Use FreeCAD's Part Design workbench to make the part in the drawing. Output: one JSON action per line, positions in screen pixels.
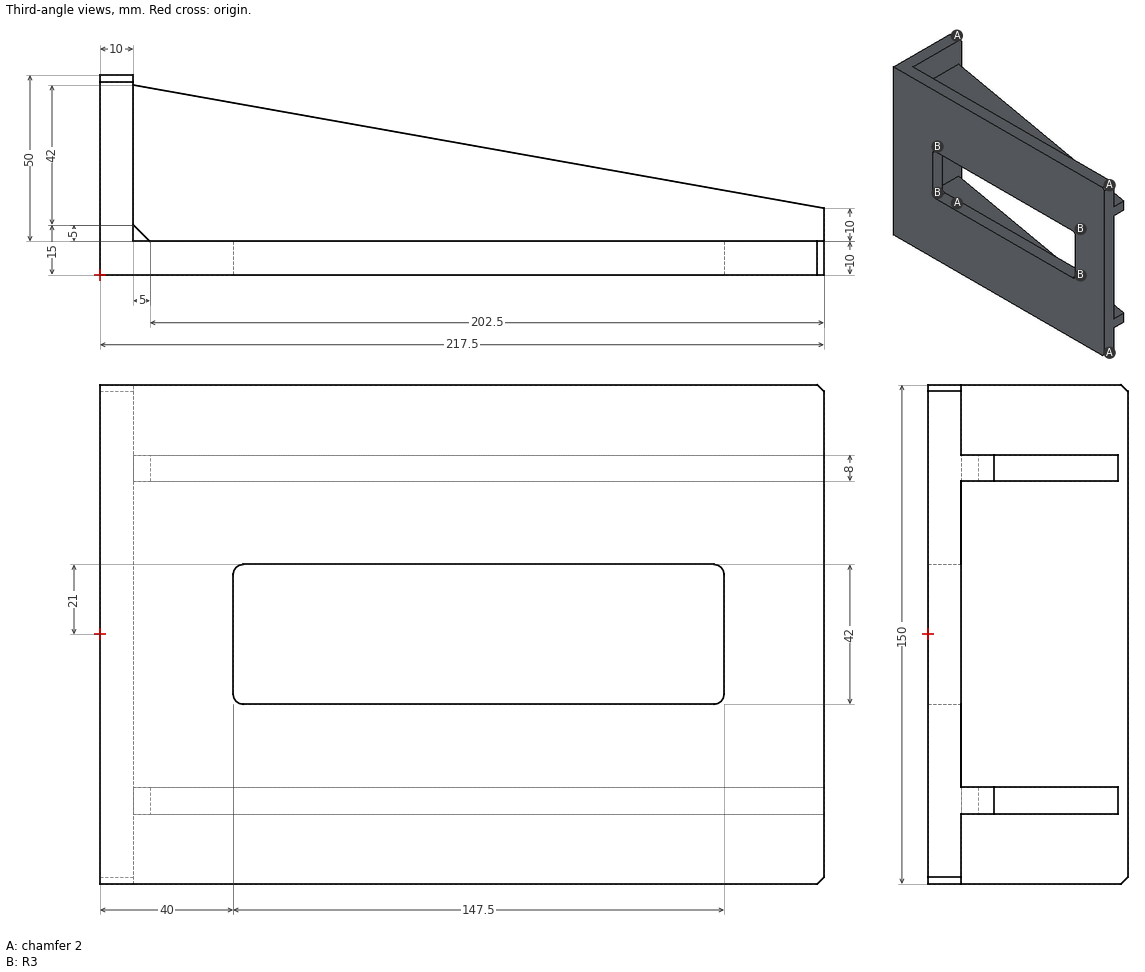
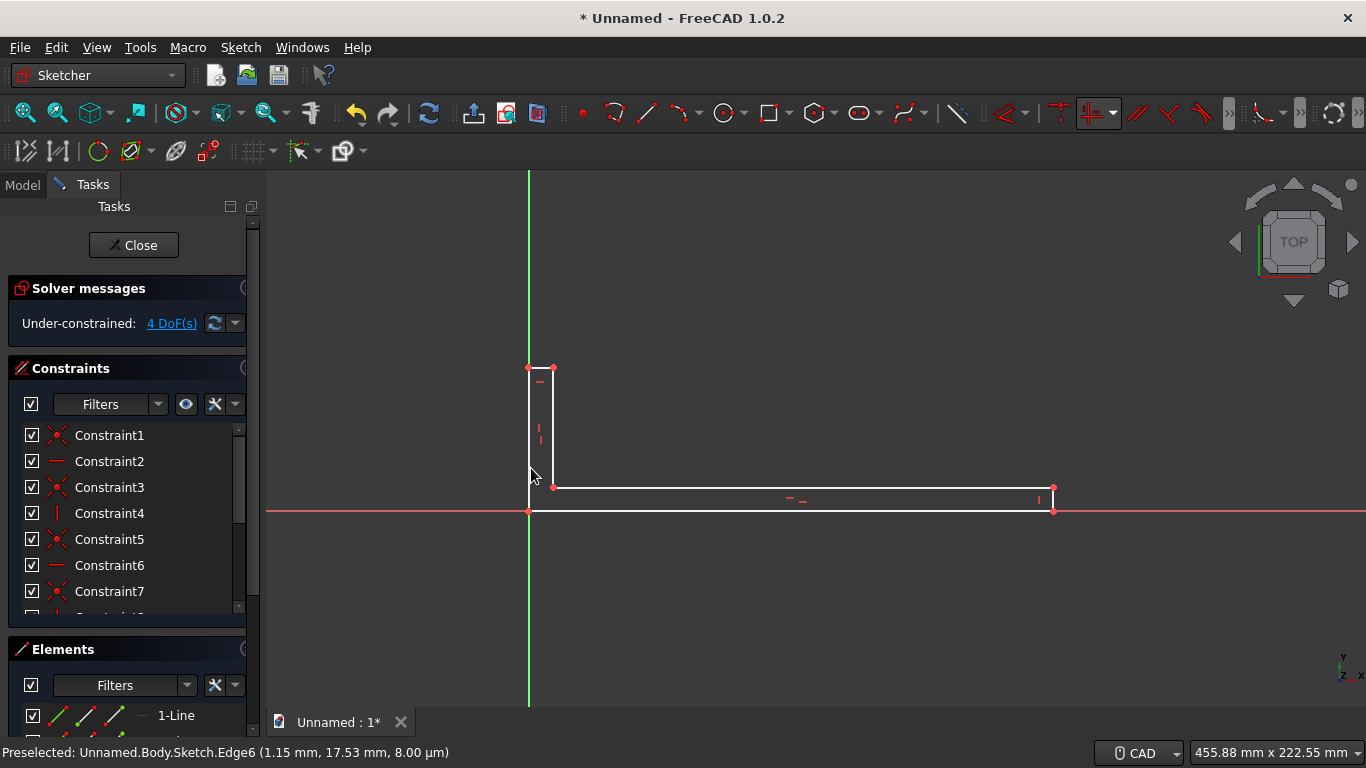
{"action": "left_click", "coordinate": [1004, 114]}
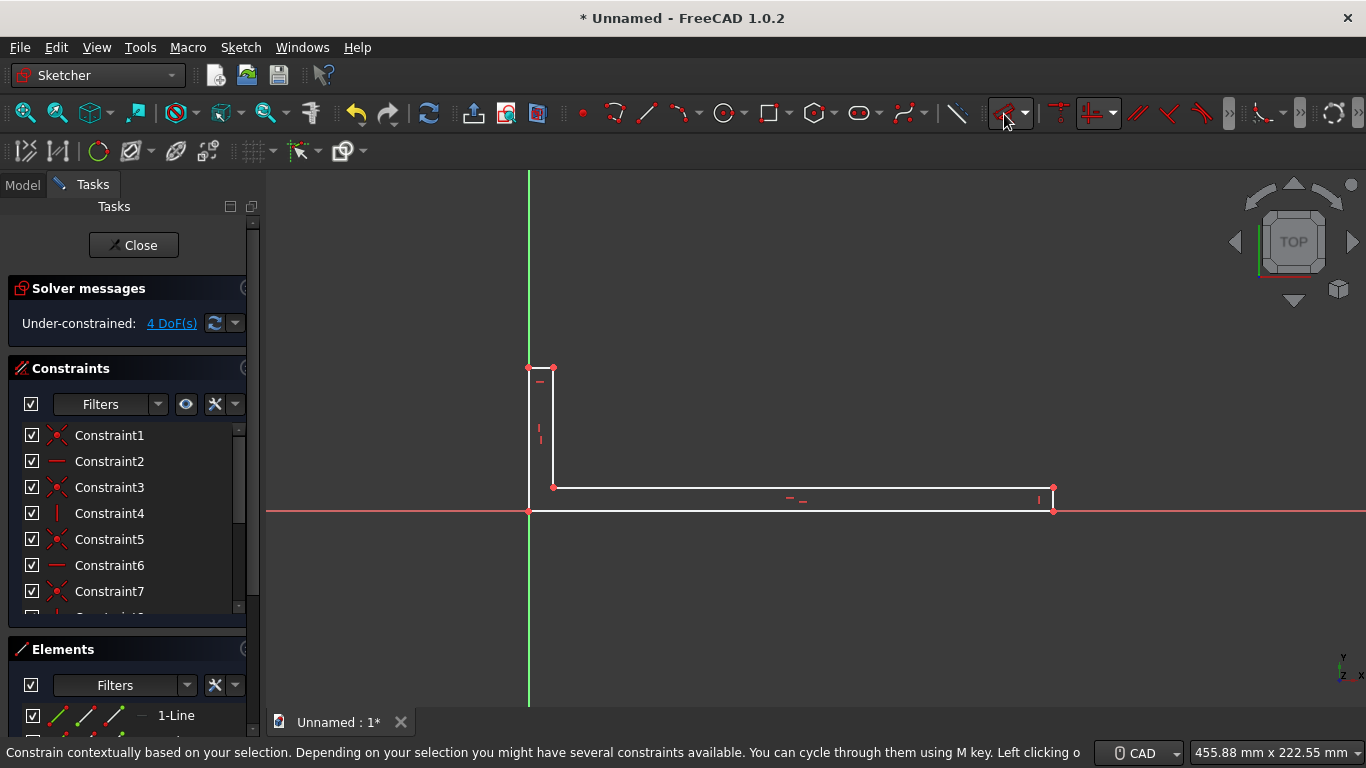
{"action": "scroll", "coordinate": [1053, 502], "scroll_direction": "up", "scroll_amount": 3}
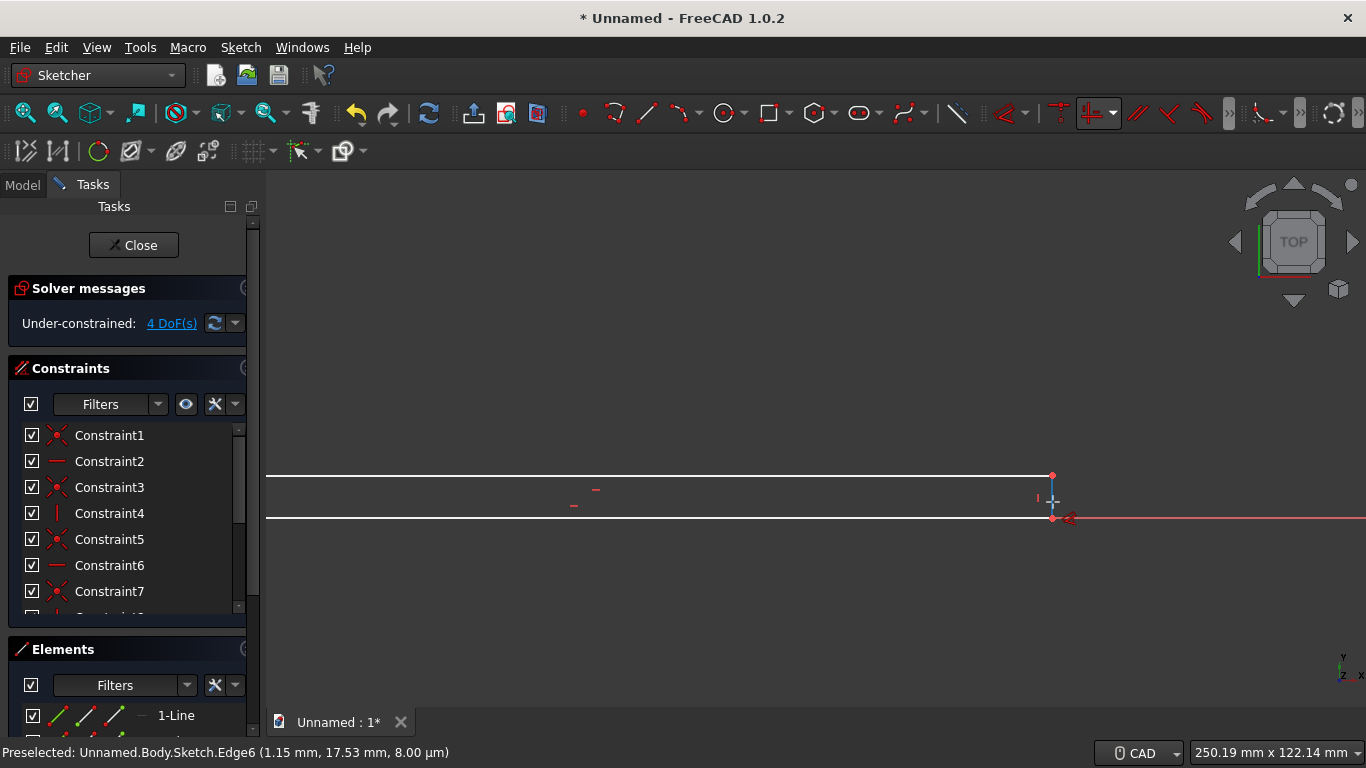
{"action": "left_click", "coordinate": [1052, 501]}
{"action": "left_click", "coordinate": [1086, 497]}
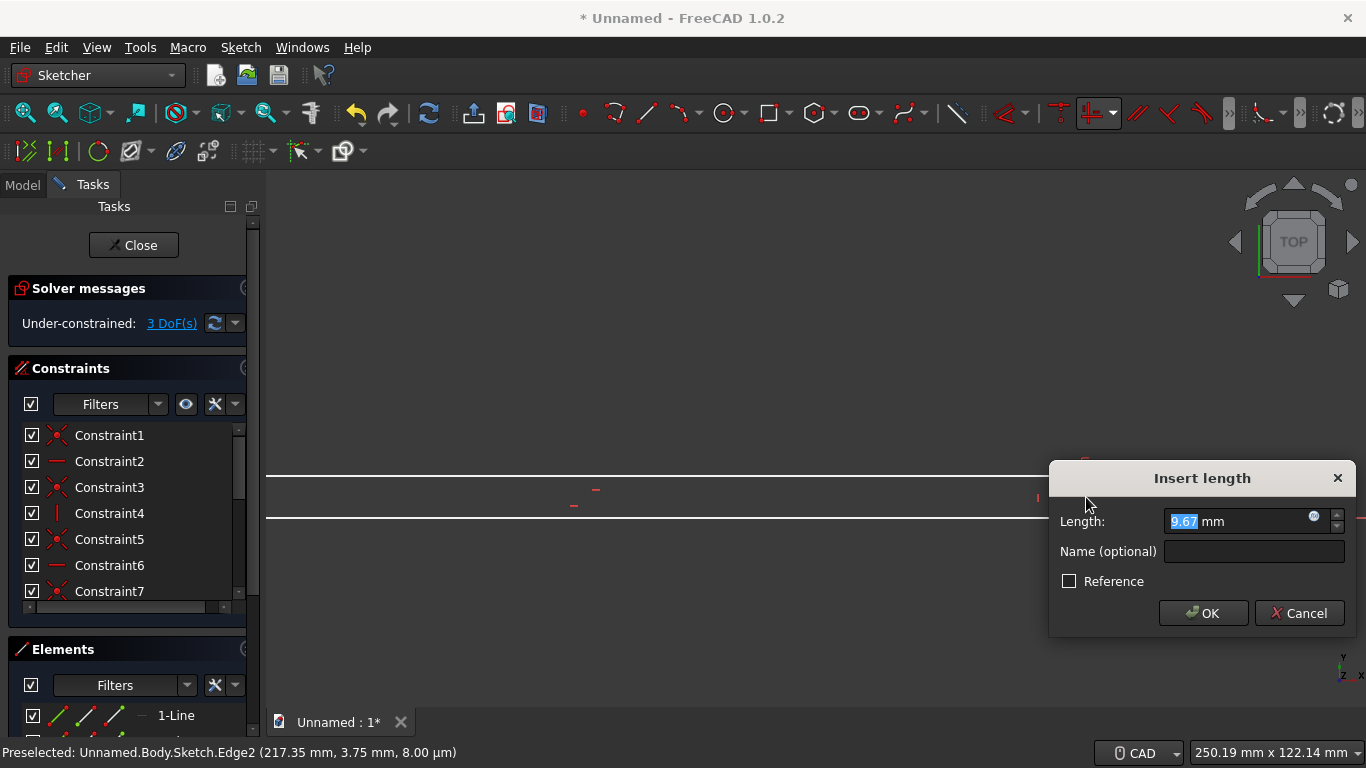
{"action": "type", "text": "10"}
{"action": "key", "text": "Return"}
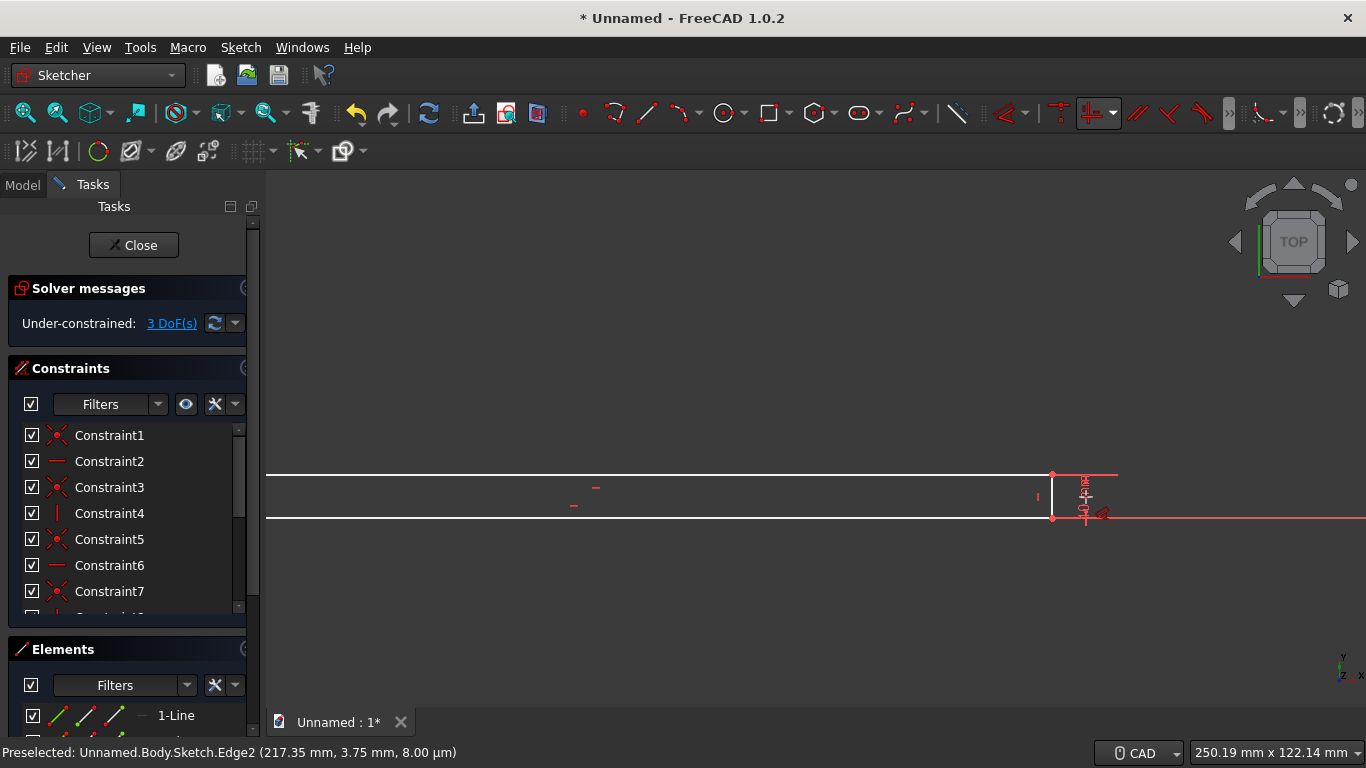
{"action": "scroll", "coordinate": [1098, 544], "scroll_direction": "down", "scroll_amount": 2}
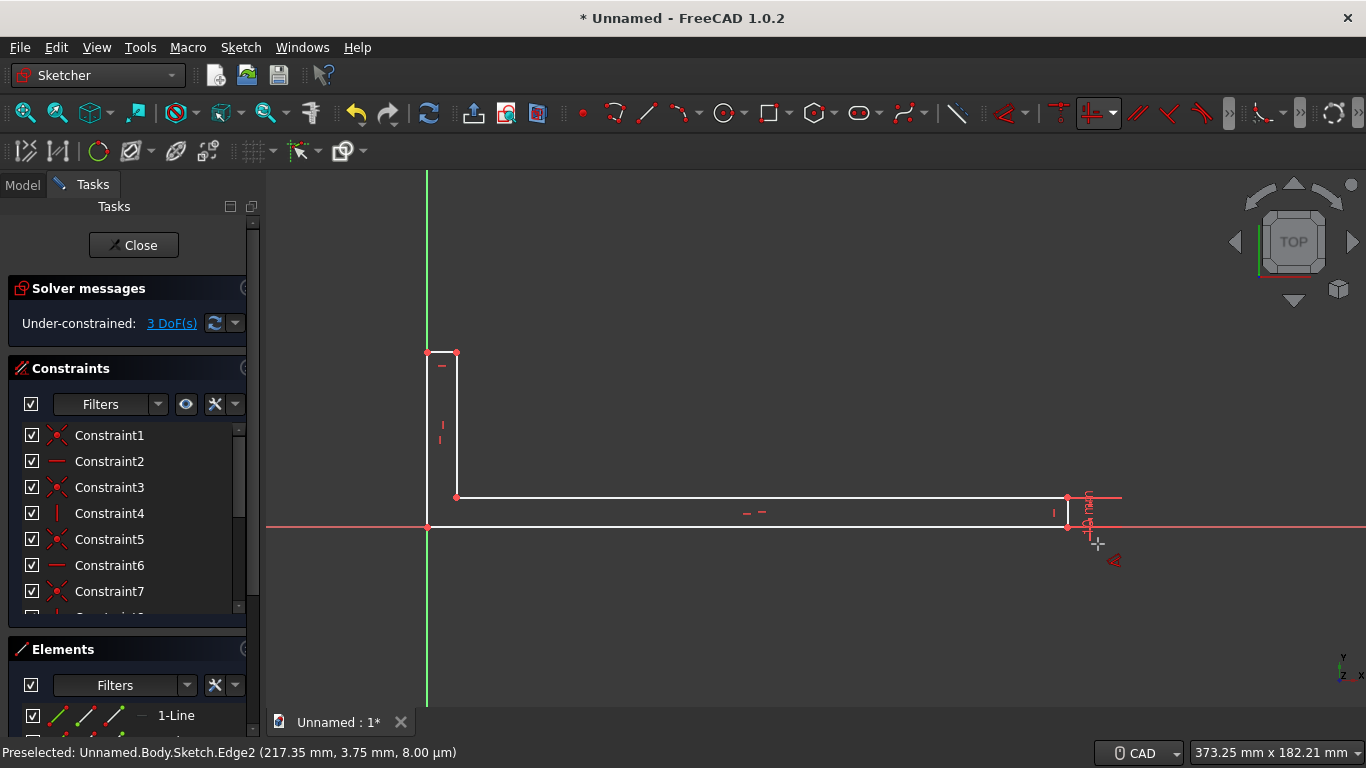
{"action": "left_click", "coordinate": [457, 454]}
{"action": "left_click", "coordinate": [491, 425]}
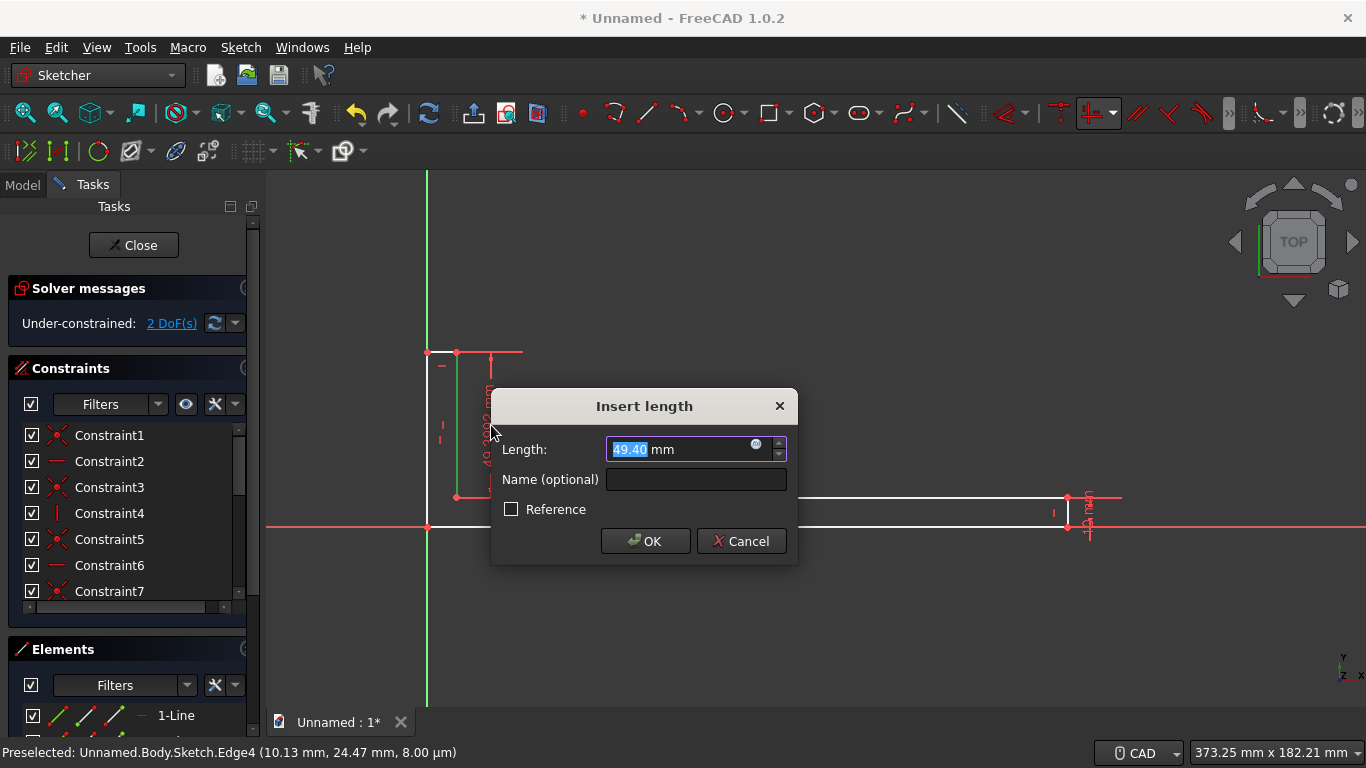
{"action": "type", "text": "50"}
{"action": "key", "text": "Return"}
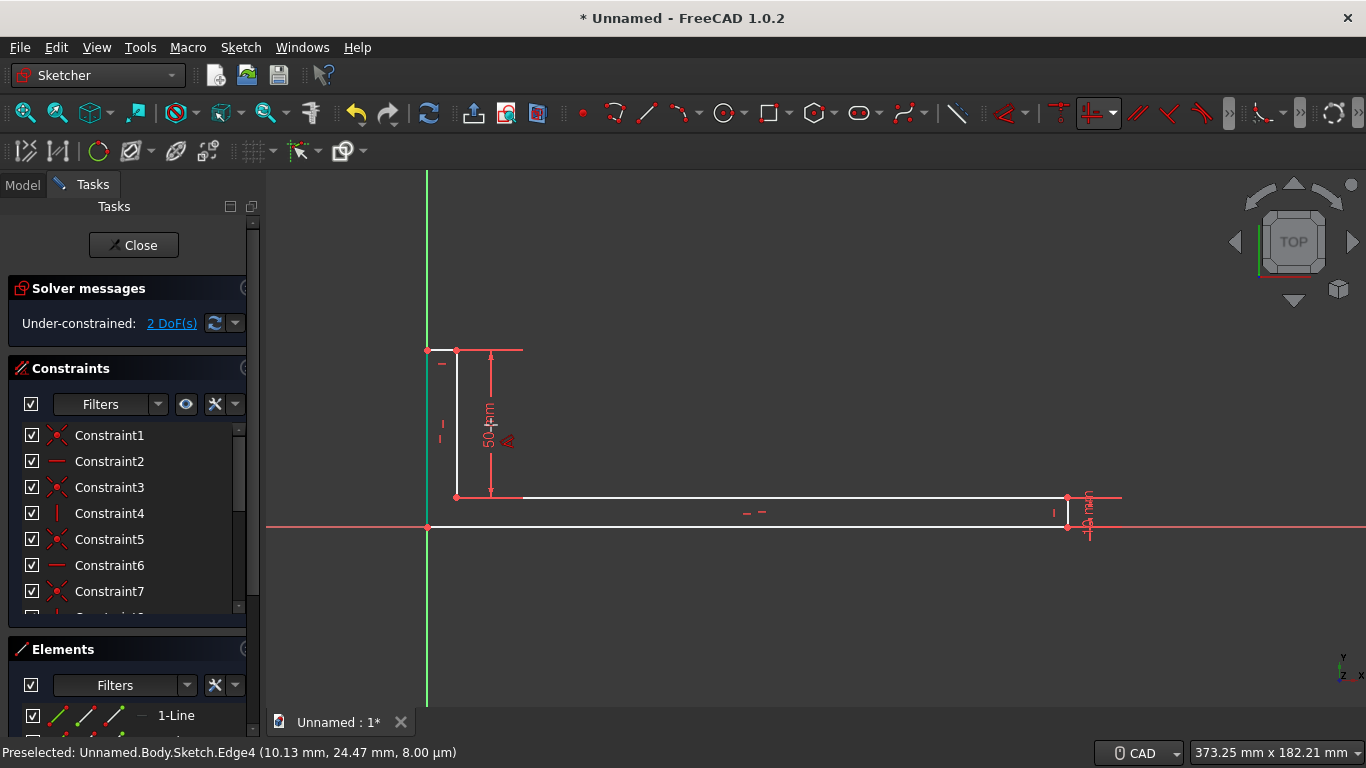
{"action": "scroll", "coordinate": [445, 350], "scroll_direction": "up", "scroll_amount": 2}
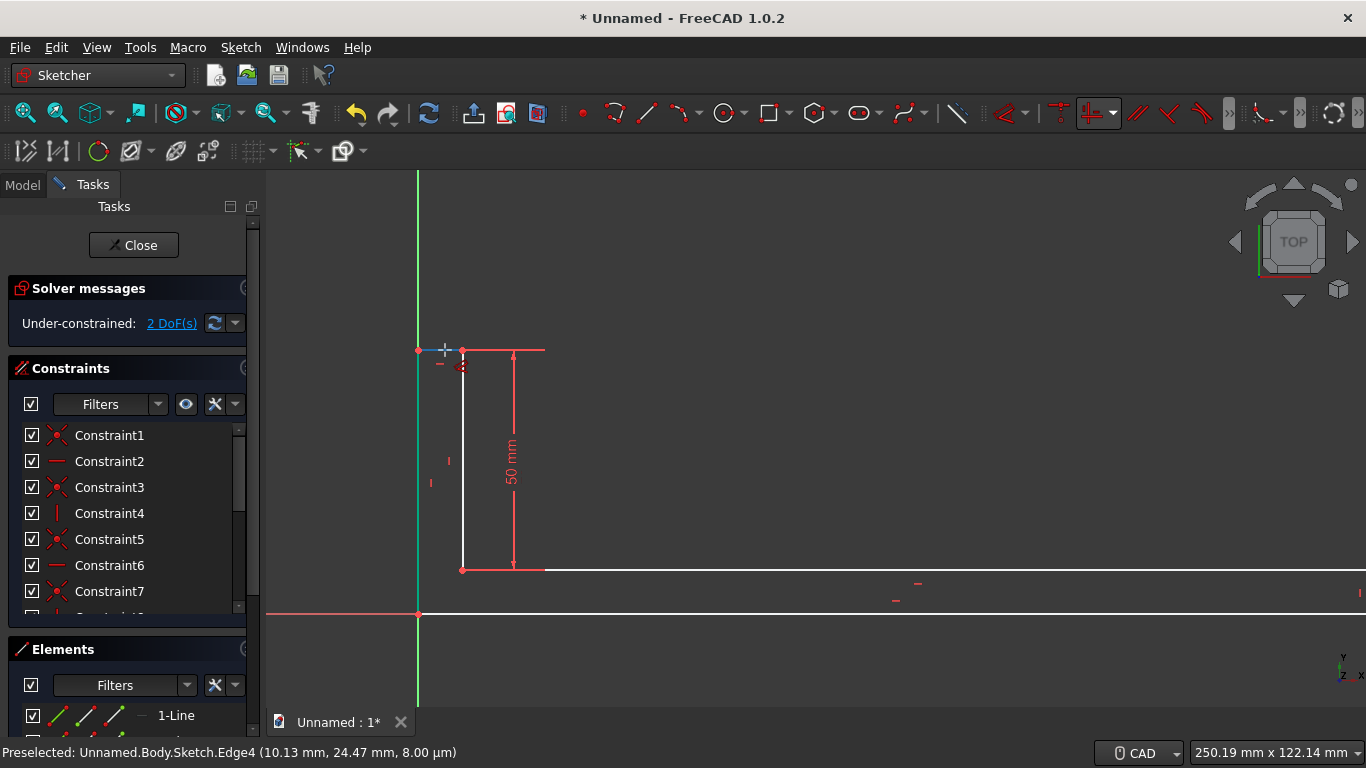
{"action": "left_click", "coordinate": [445, 350]}
{"action": "left_click", "coordinate": [441, 316]}